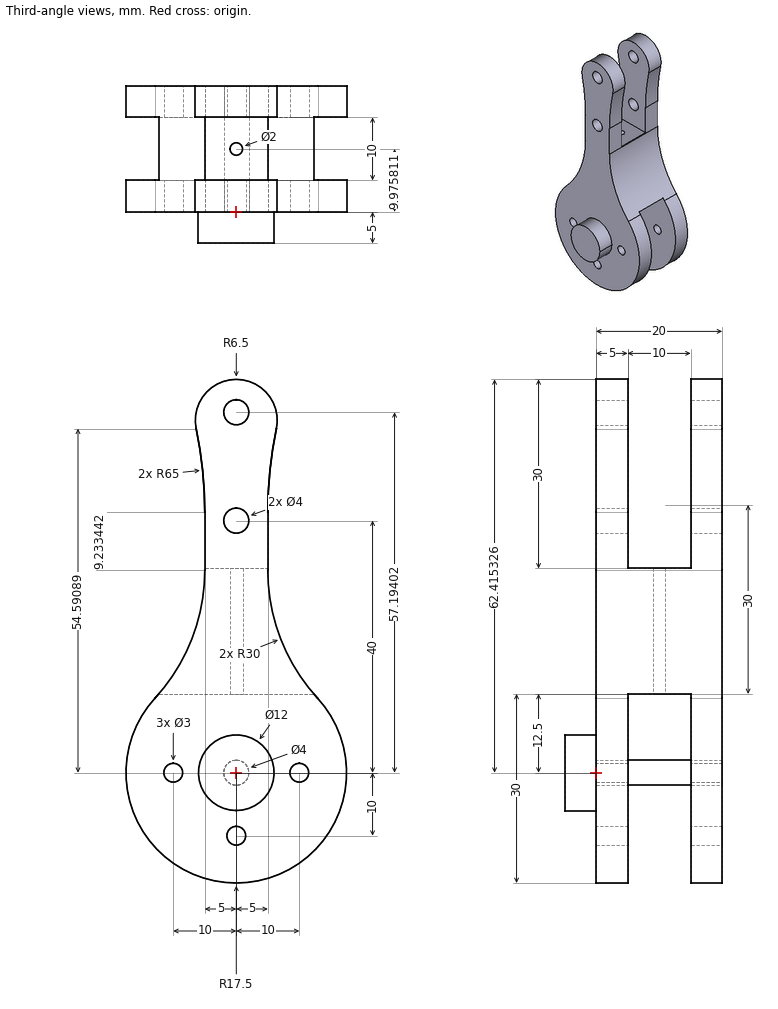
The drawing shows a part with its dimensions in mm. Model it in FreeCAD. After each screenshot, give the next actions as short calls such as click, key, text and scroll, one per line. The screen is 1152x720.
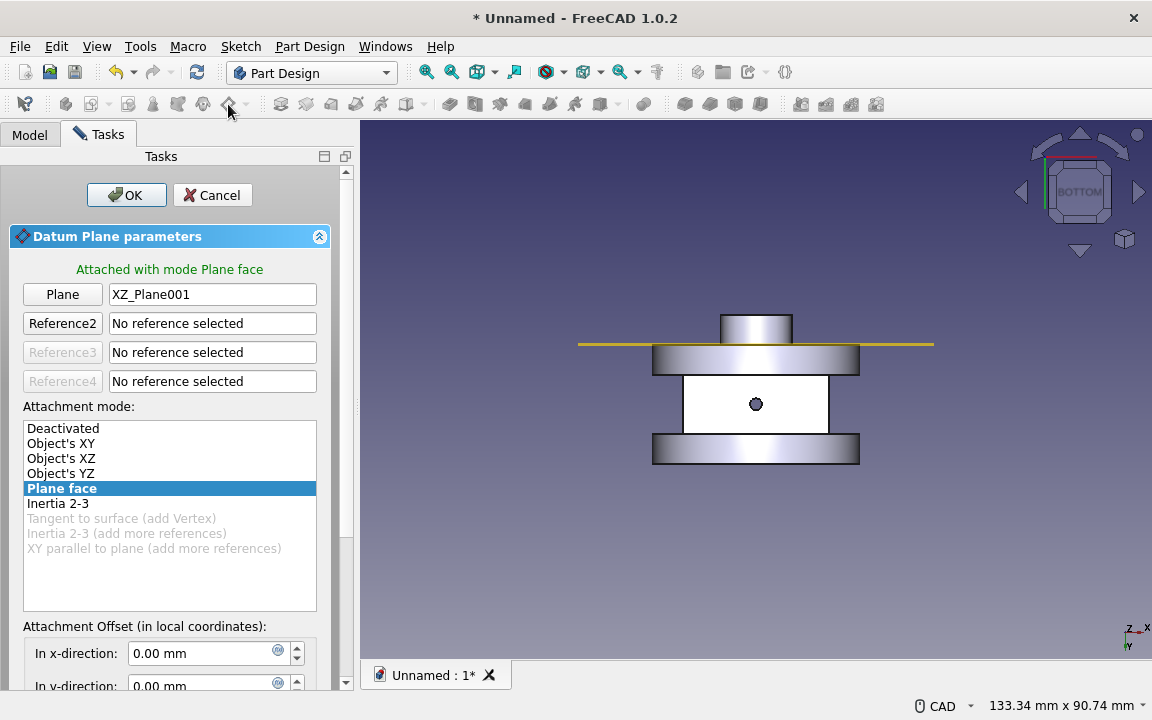
scroll(346, 428, down, 2)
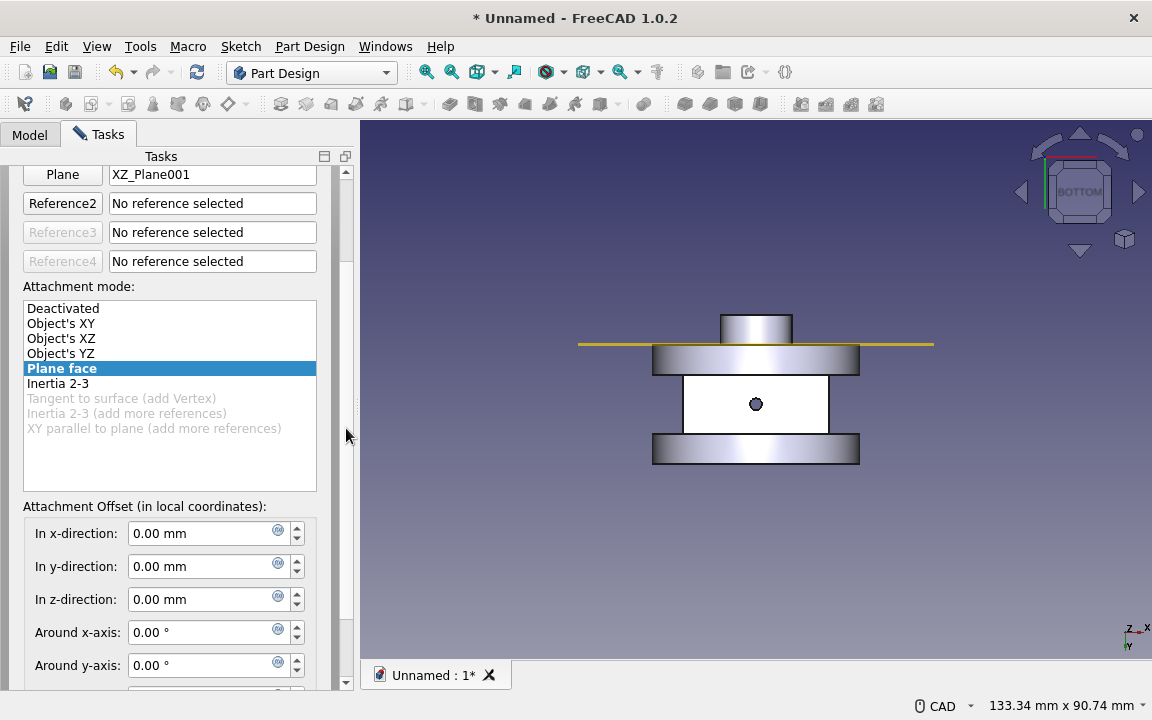
triple_click(210, 600)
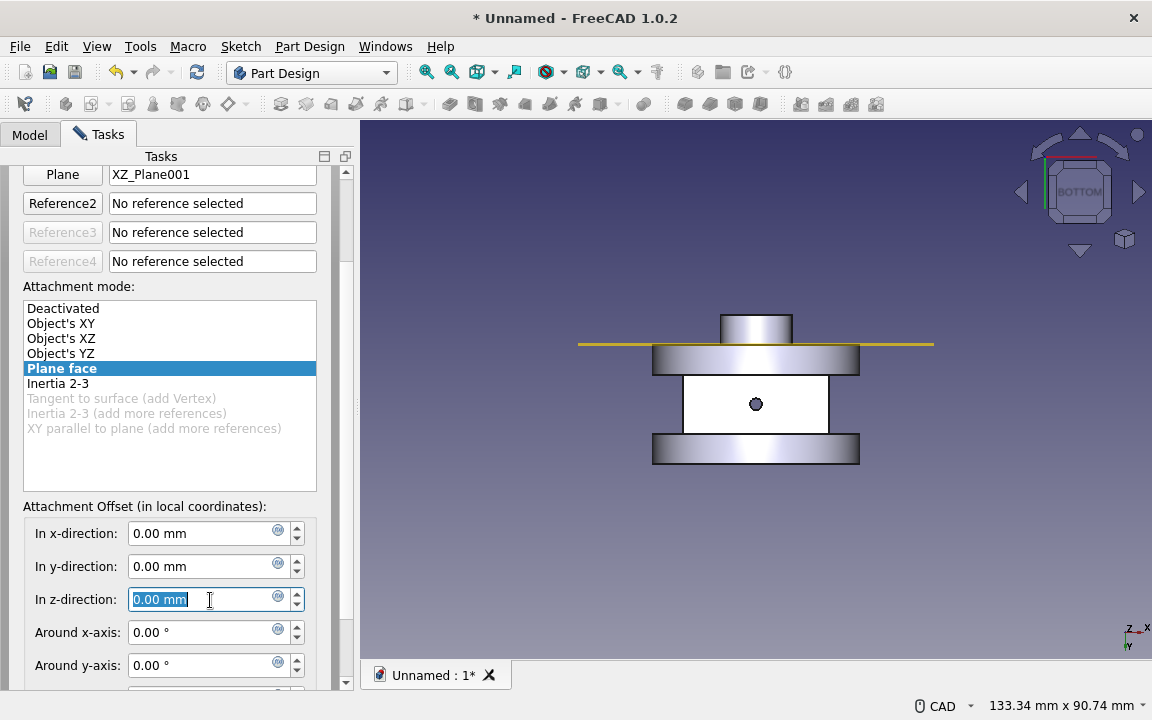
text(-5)
key(Tab)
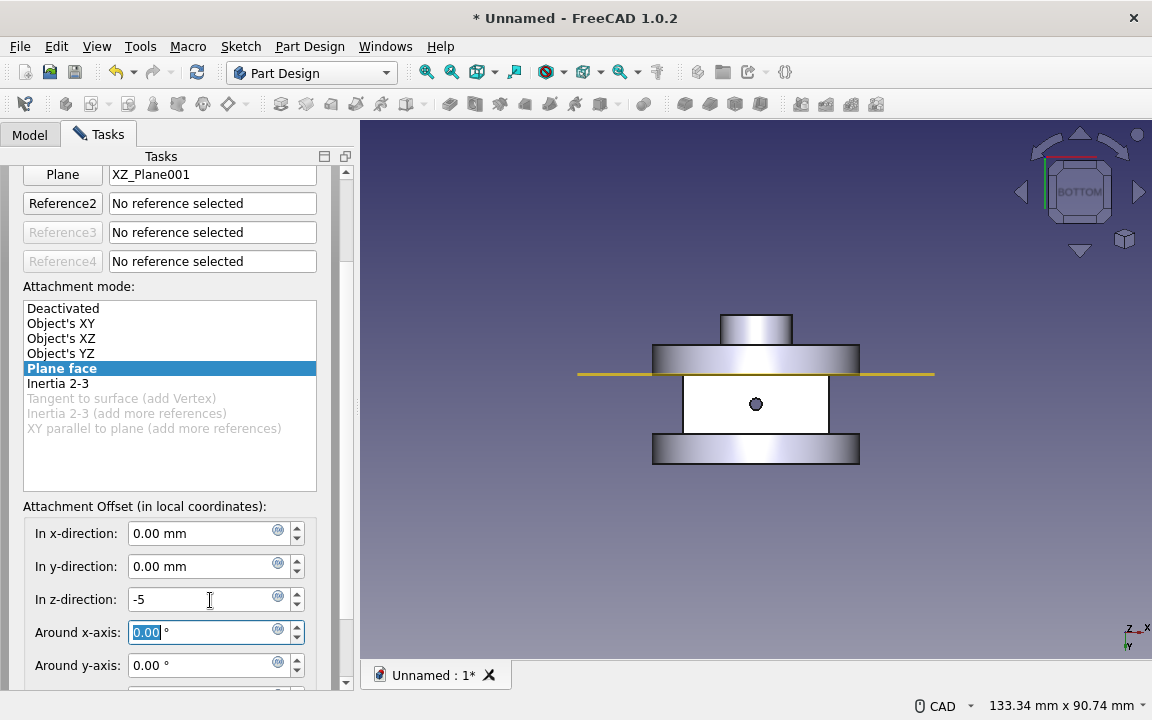
scroll(346, 428, up, 3)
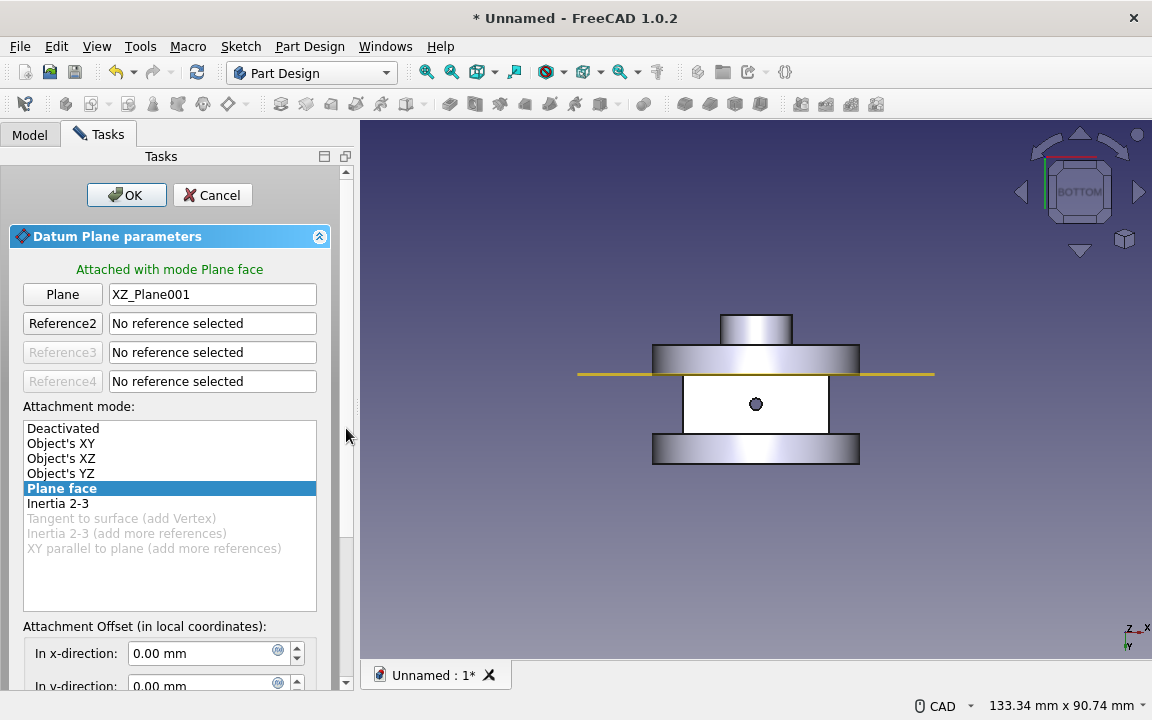
click(127, 195)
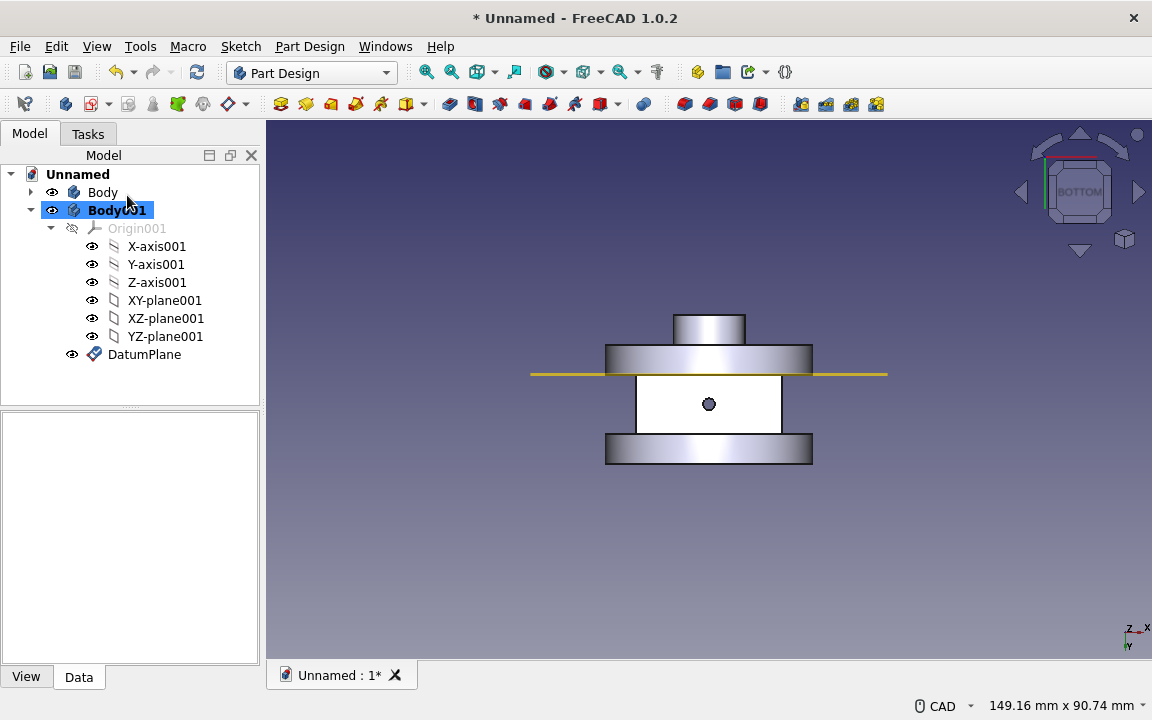
click(117, 354)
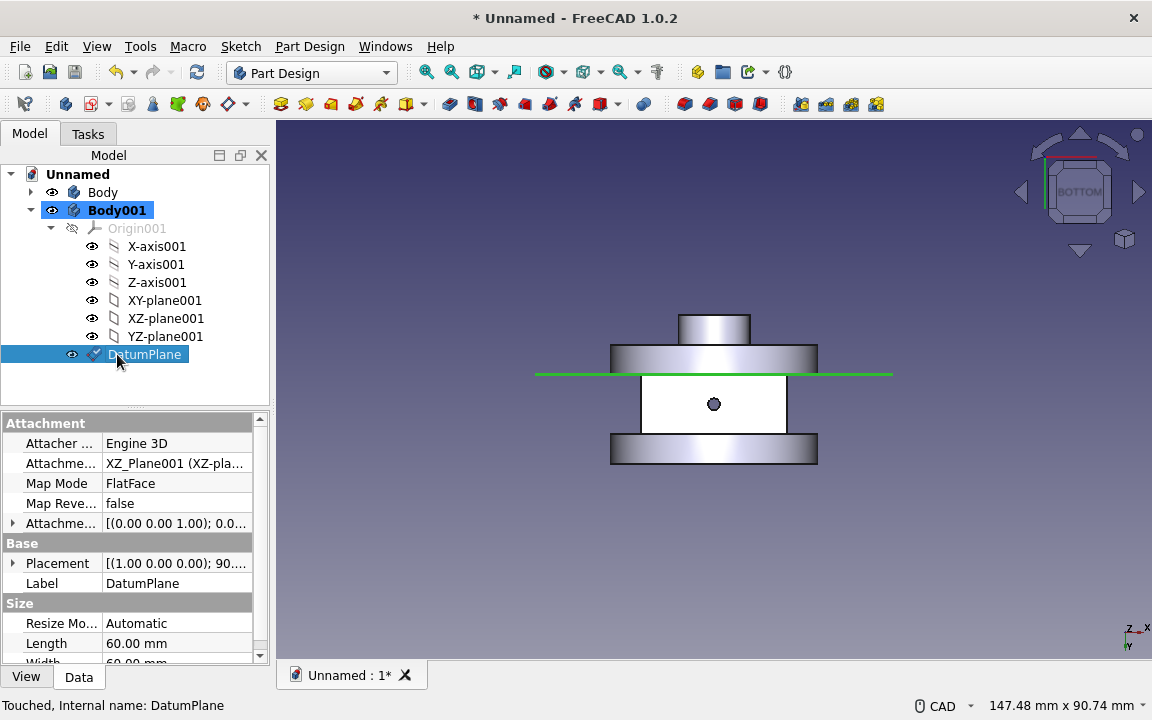
click(90, 104)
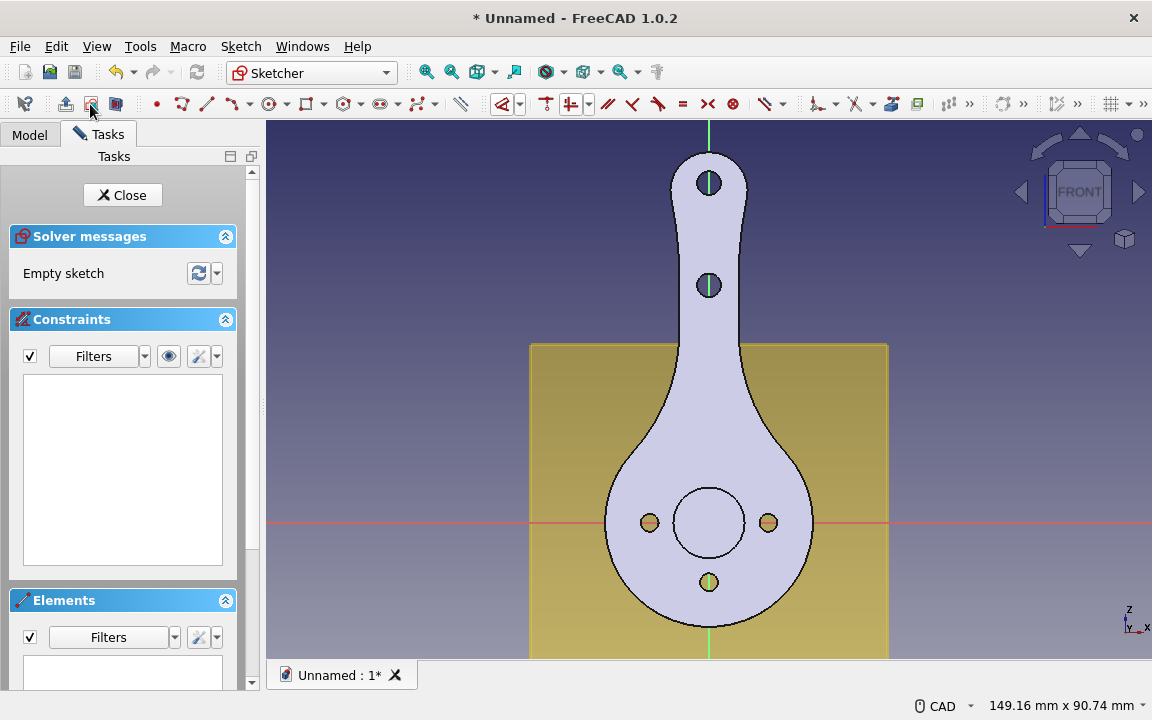
scroll(714, 534, up, 13)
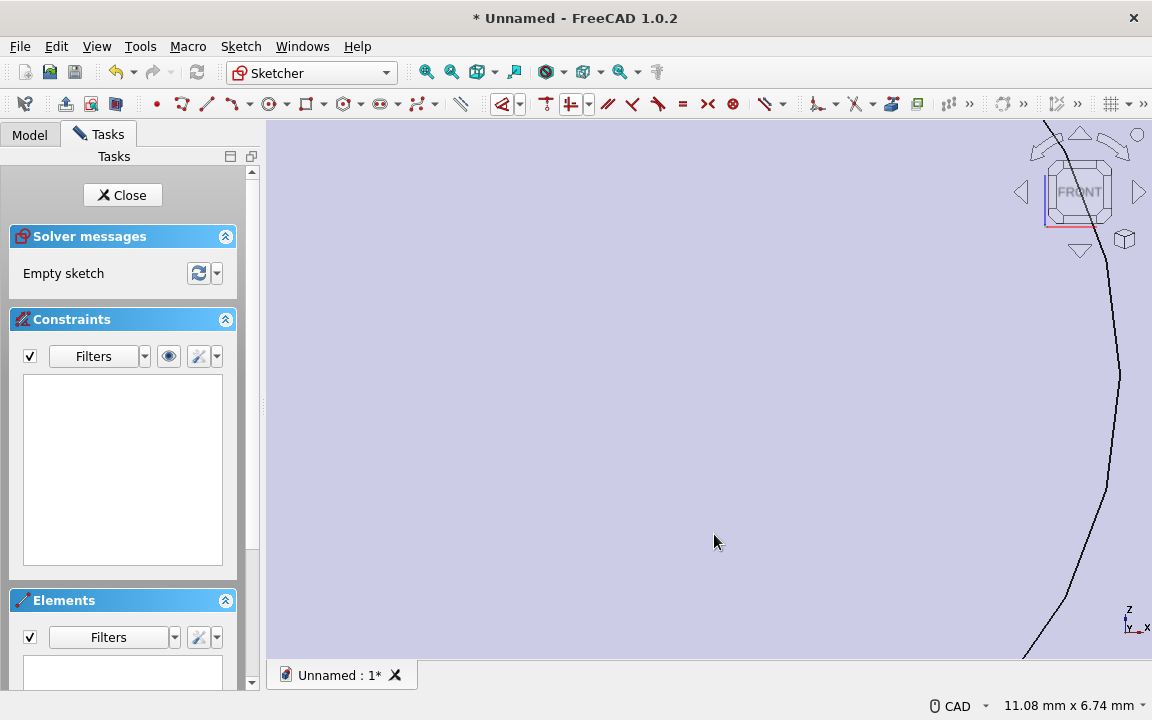
click(268, 104)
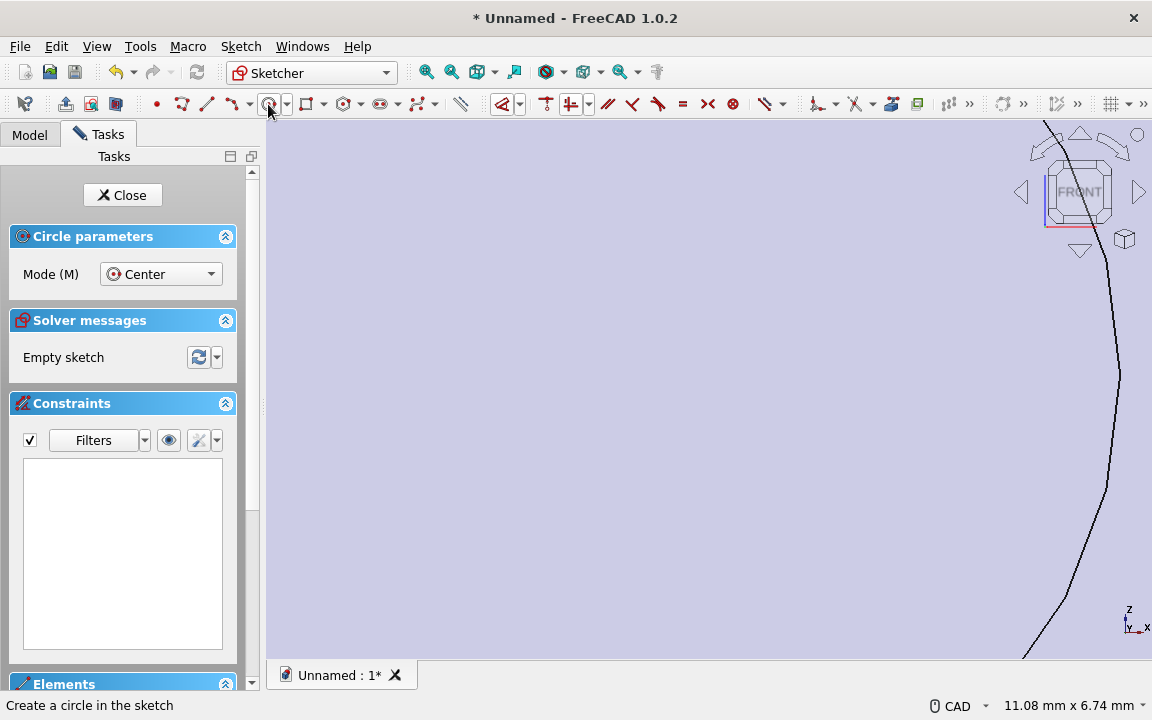
click(640, 375)
click(753, 262)
key(Escape)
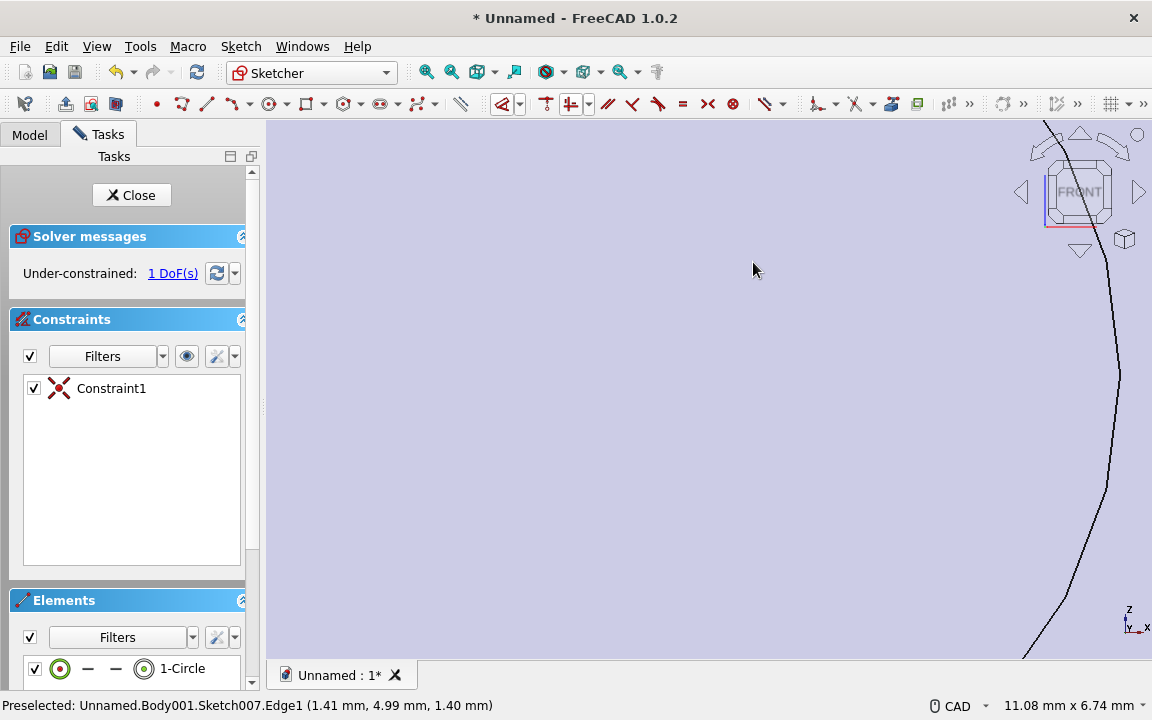
click(752, 262)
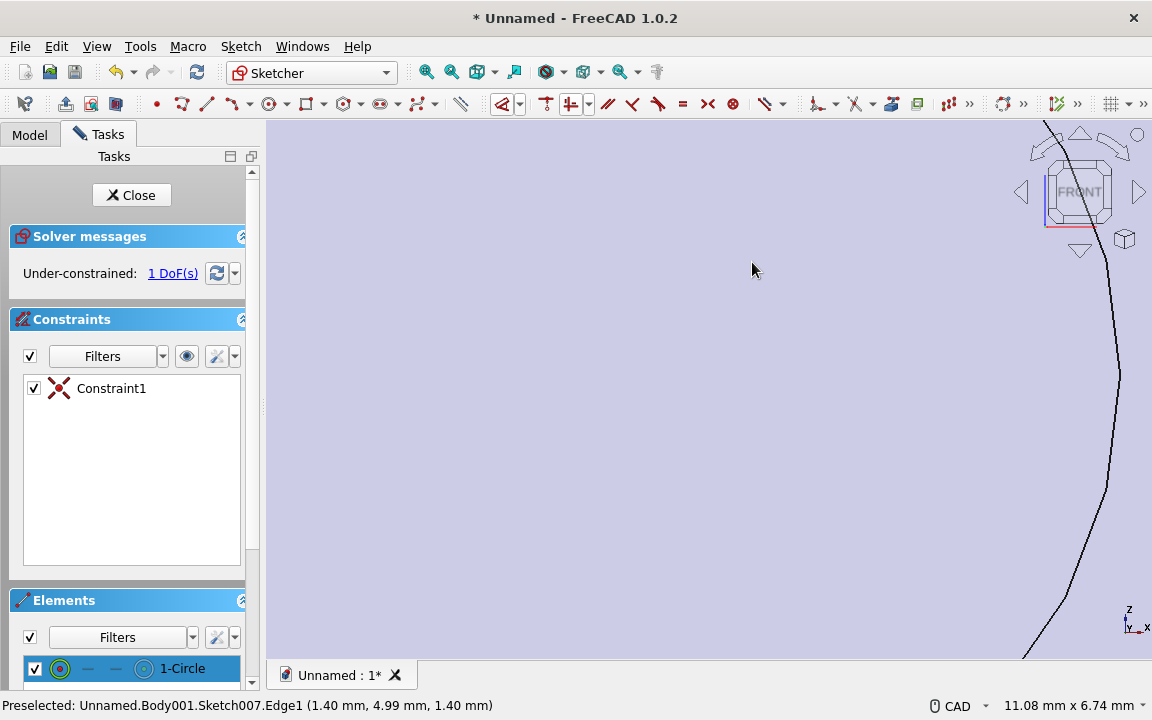
click(520, 104)